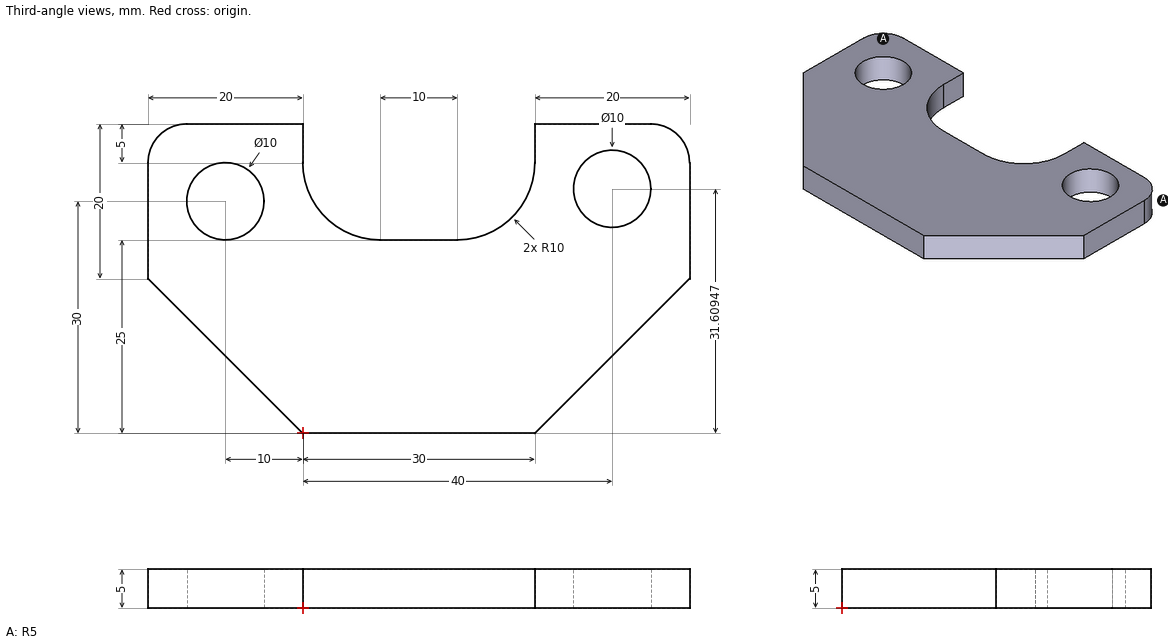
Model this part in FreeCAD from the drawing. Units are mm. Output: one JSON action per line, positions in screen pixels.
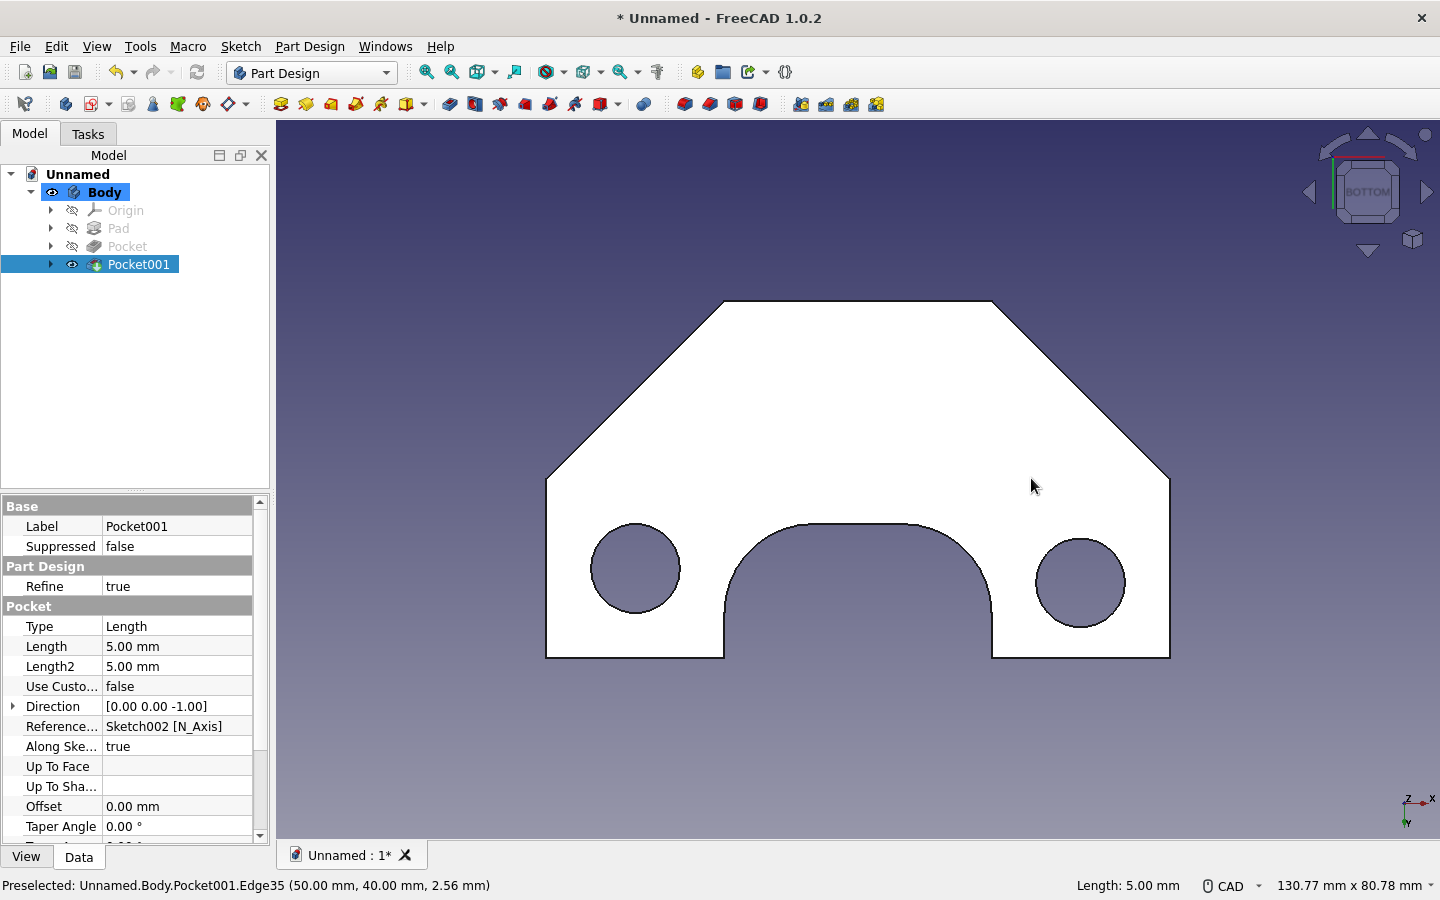
{"action": "key", "text": "4"}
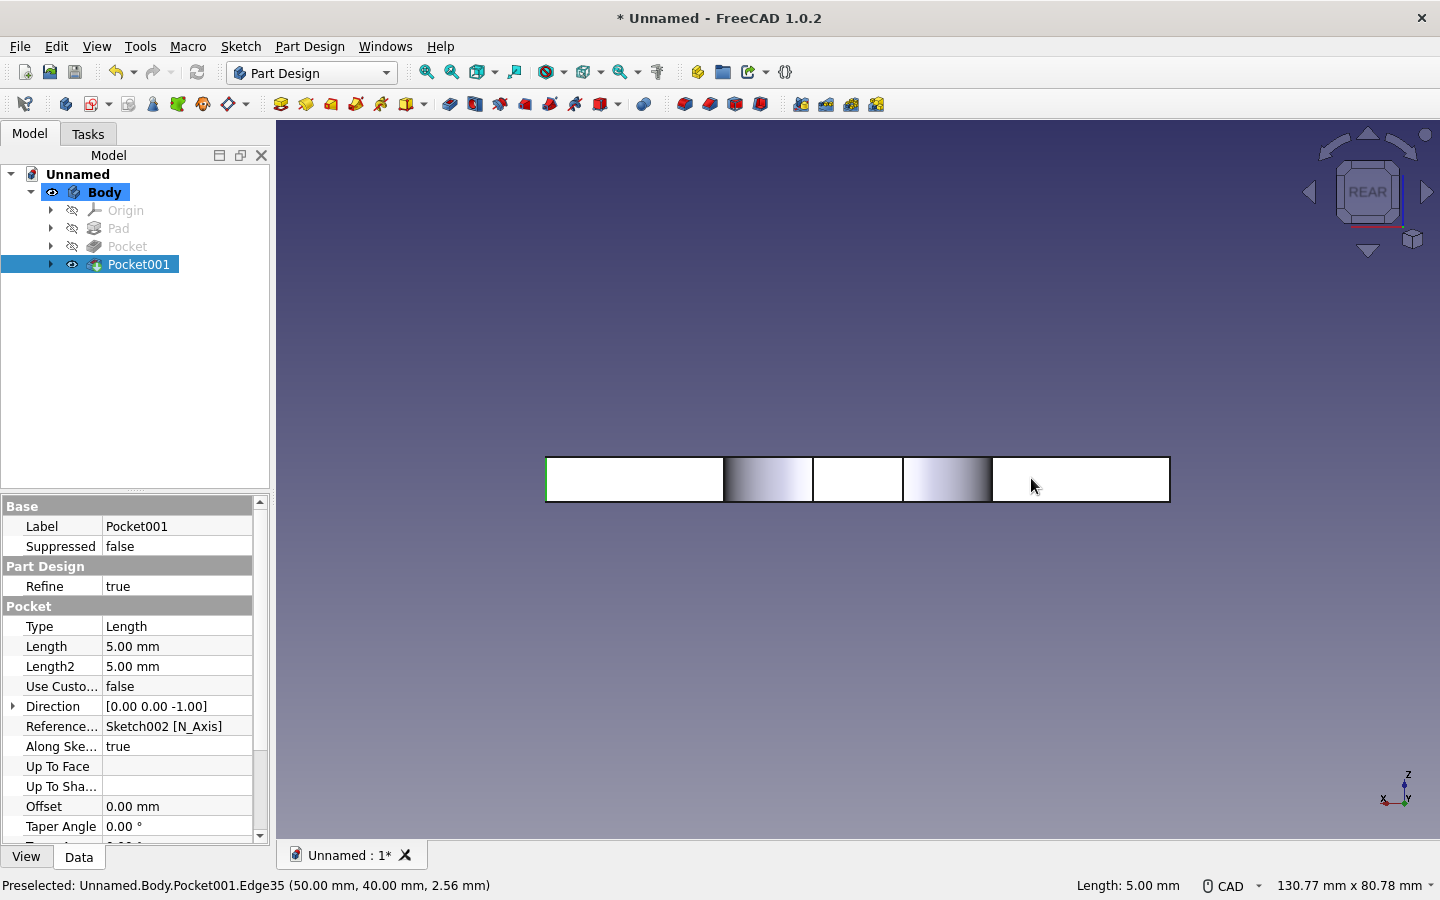
{"action": "left_click", "coordinate": [1170, 478], "text": "ctrl"}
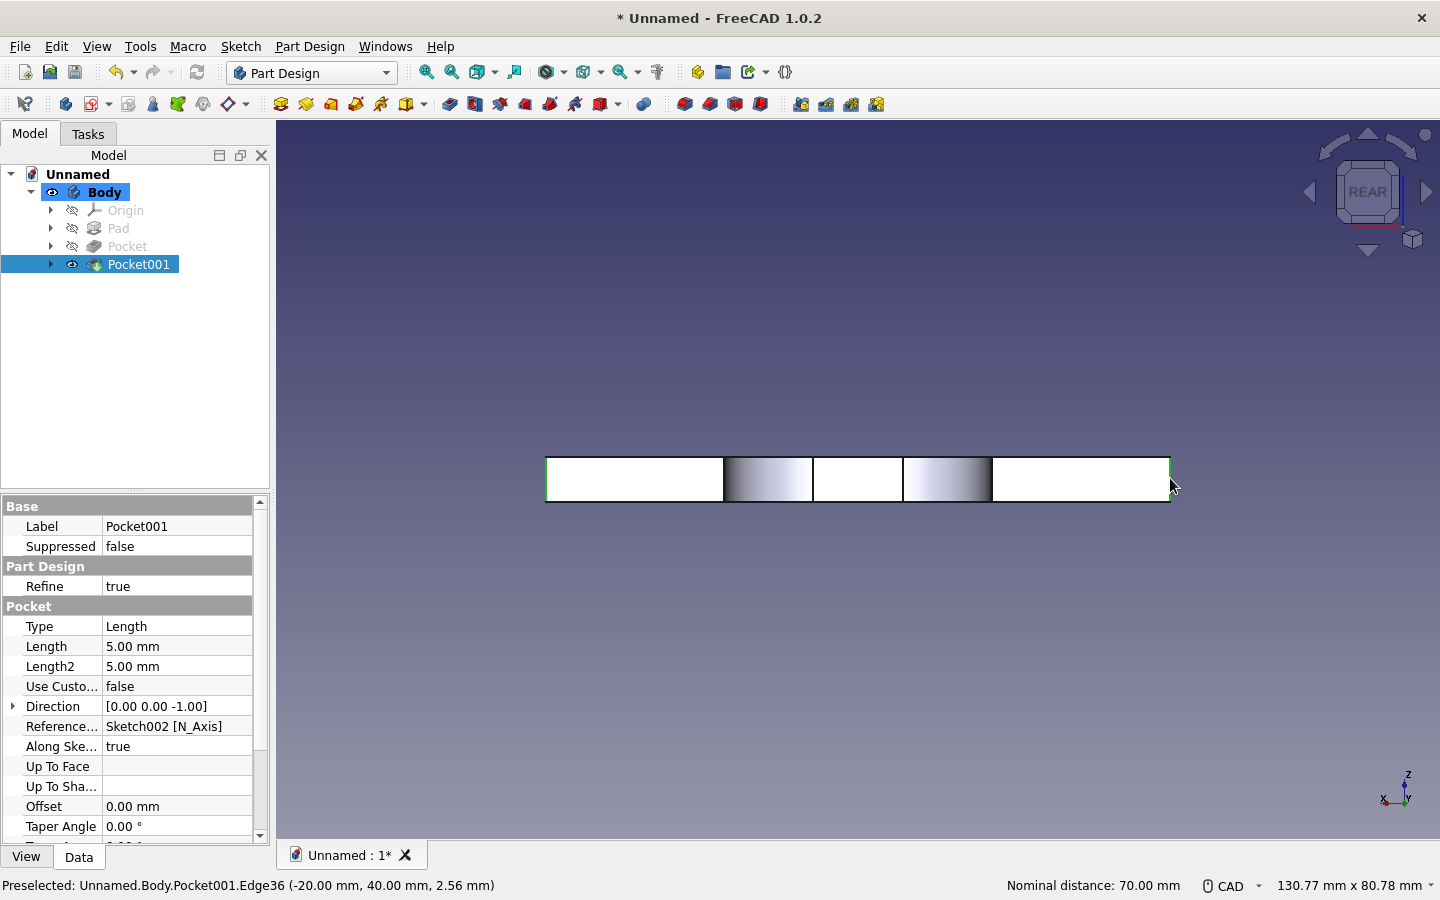
{"action": "left_click", "coordinate": [685, 104]}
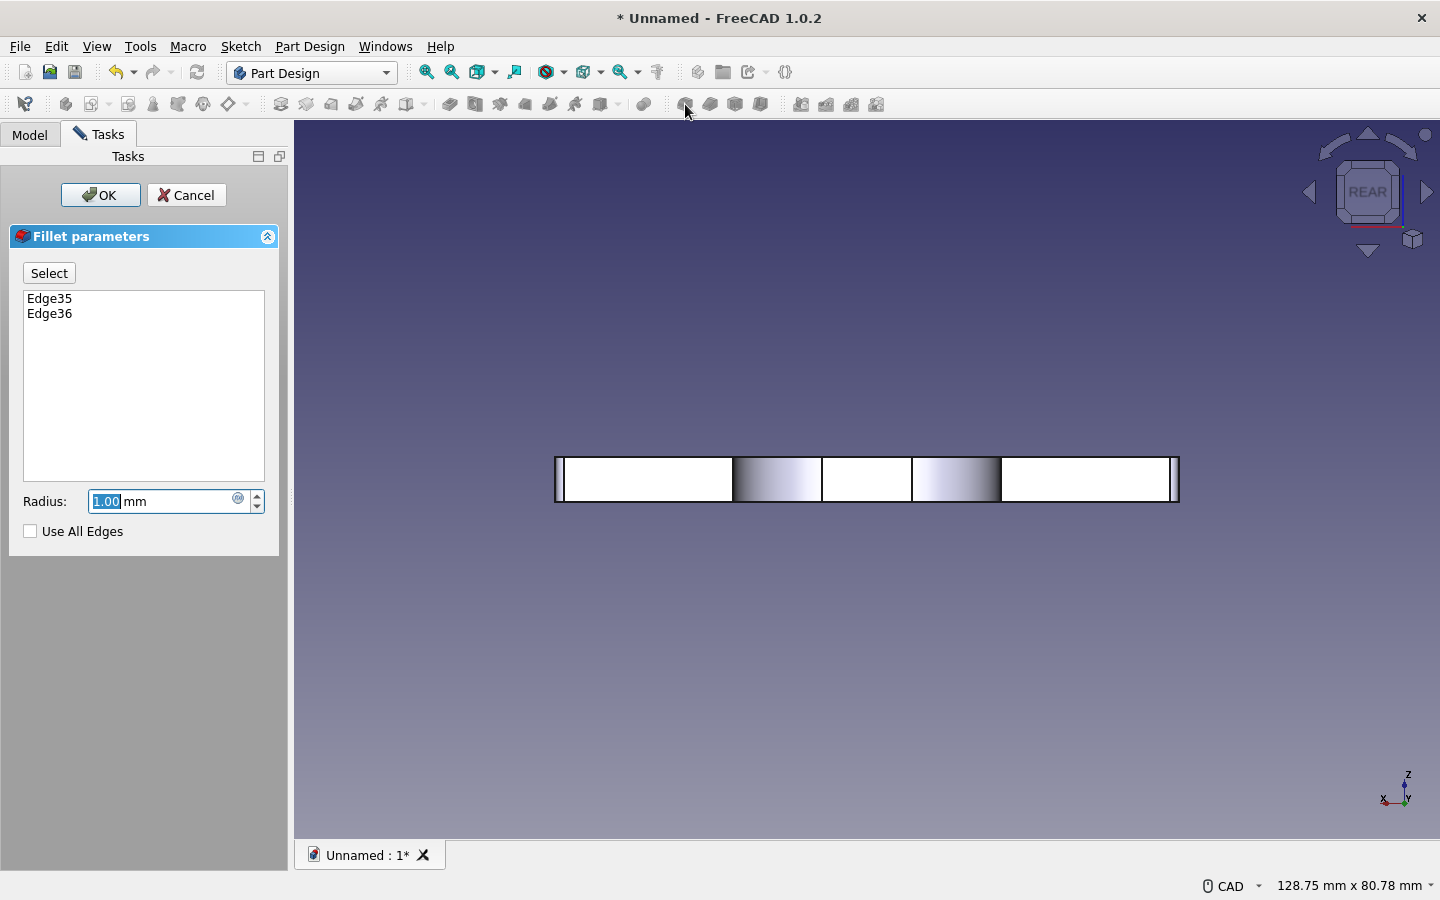
{"action": "type", "text": "5"}
{"action": "key", "text": "Tab"}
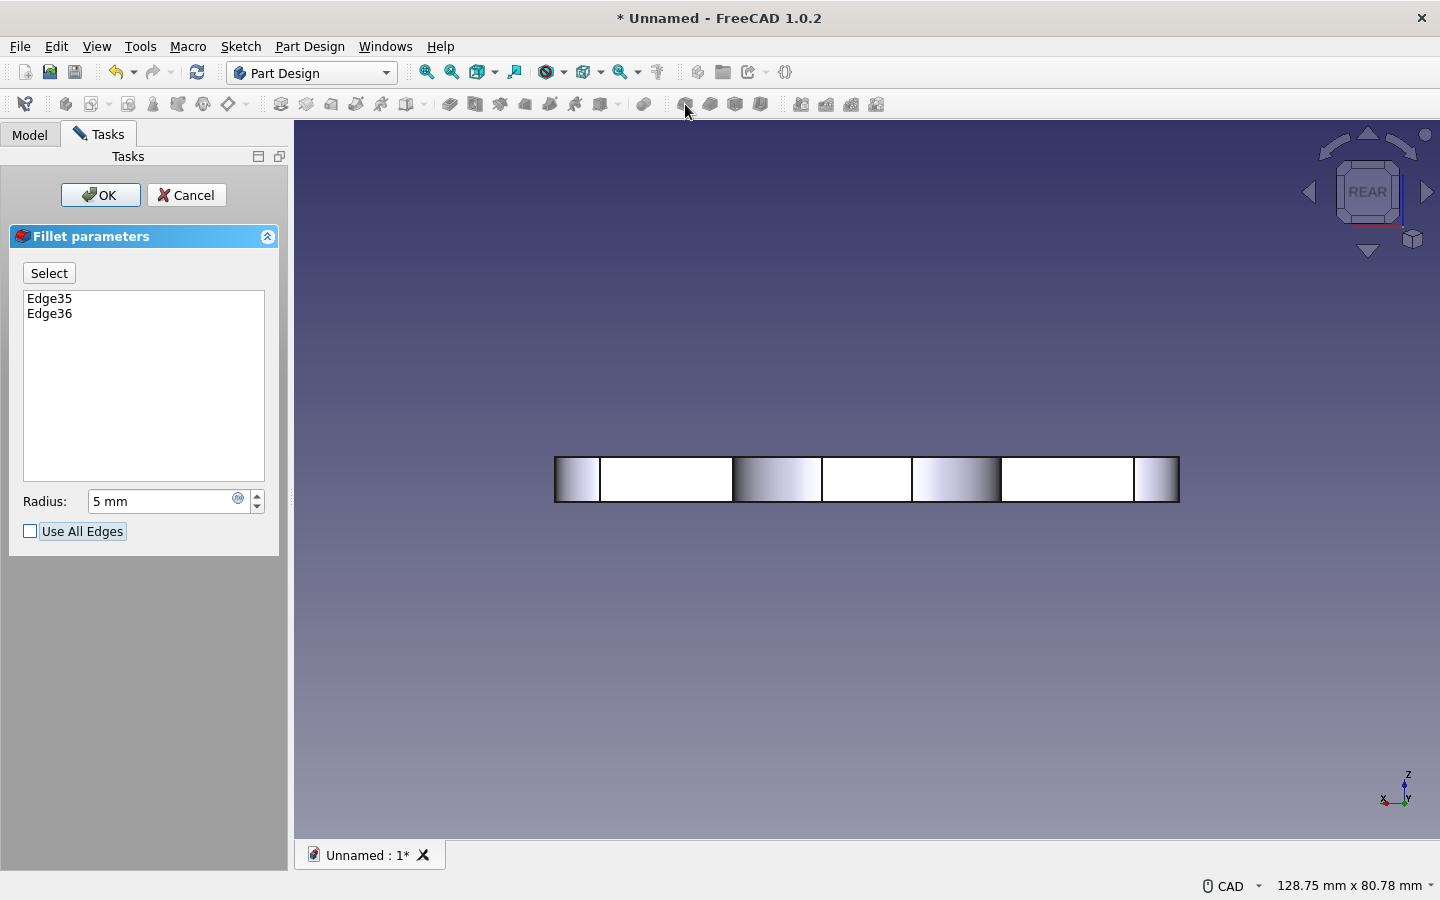
{"action": "left_click", "coordinate": [101, 195]}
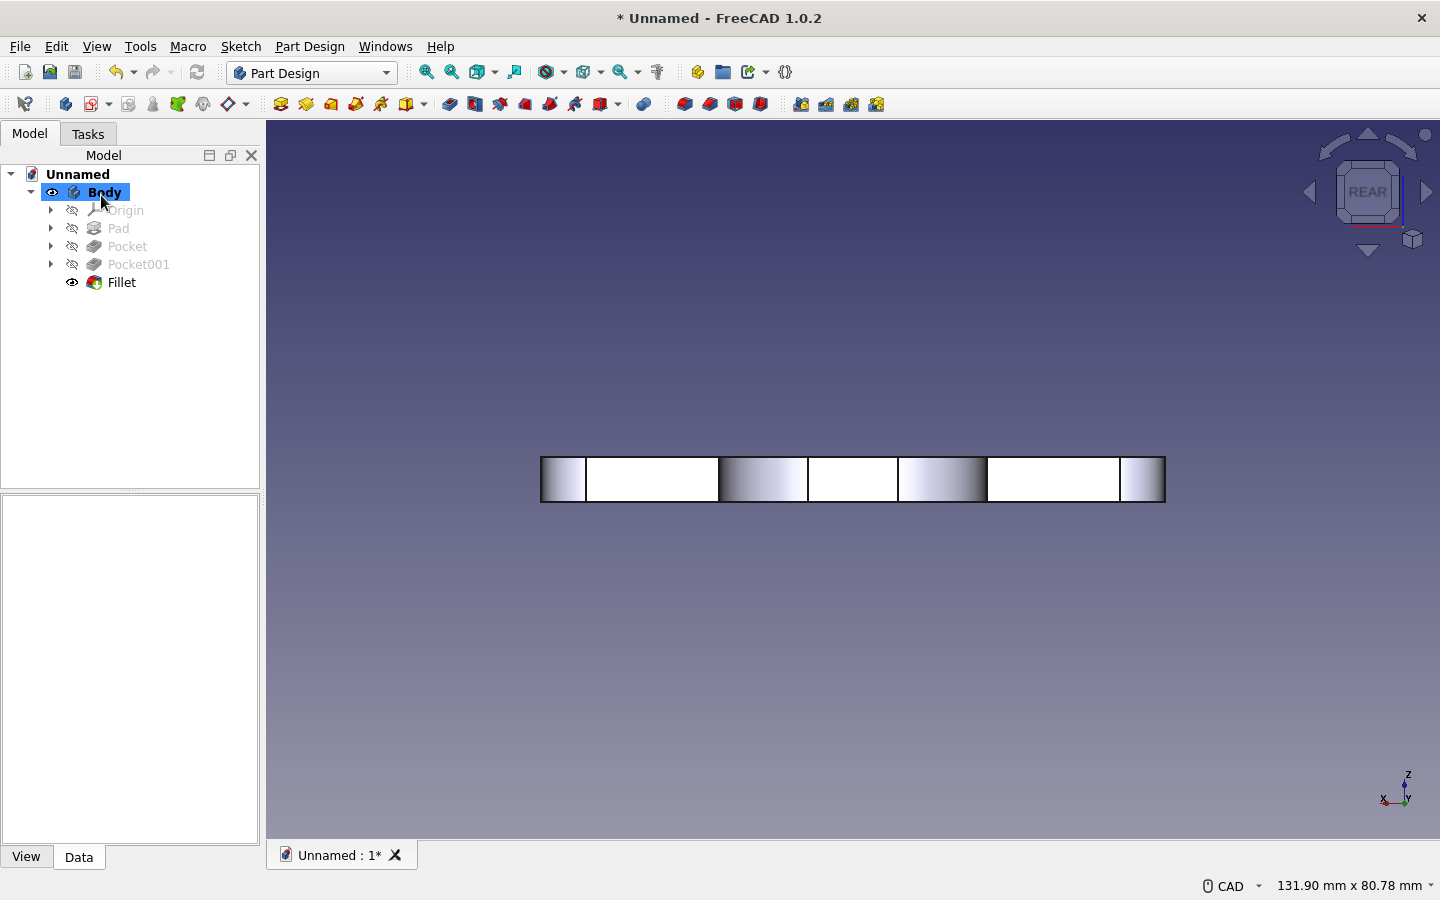
{"action": "key", "text": "0"}